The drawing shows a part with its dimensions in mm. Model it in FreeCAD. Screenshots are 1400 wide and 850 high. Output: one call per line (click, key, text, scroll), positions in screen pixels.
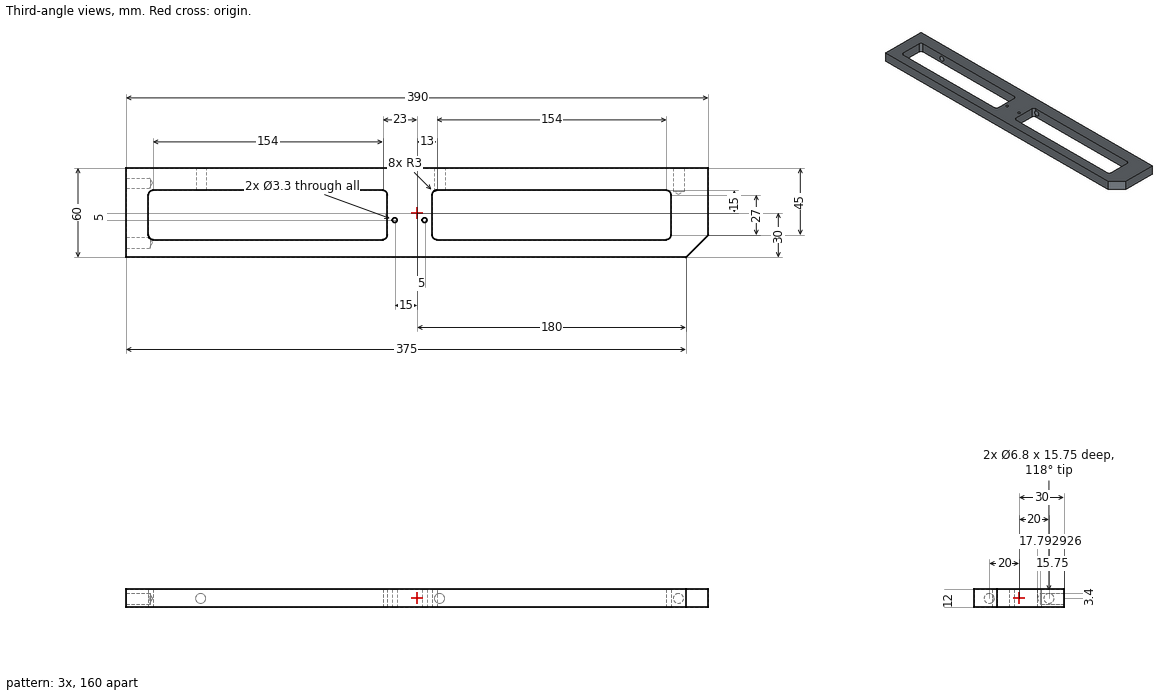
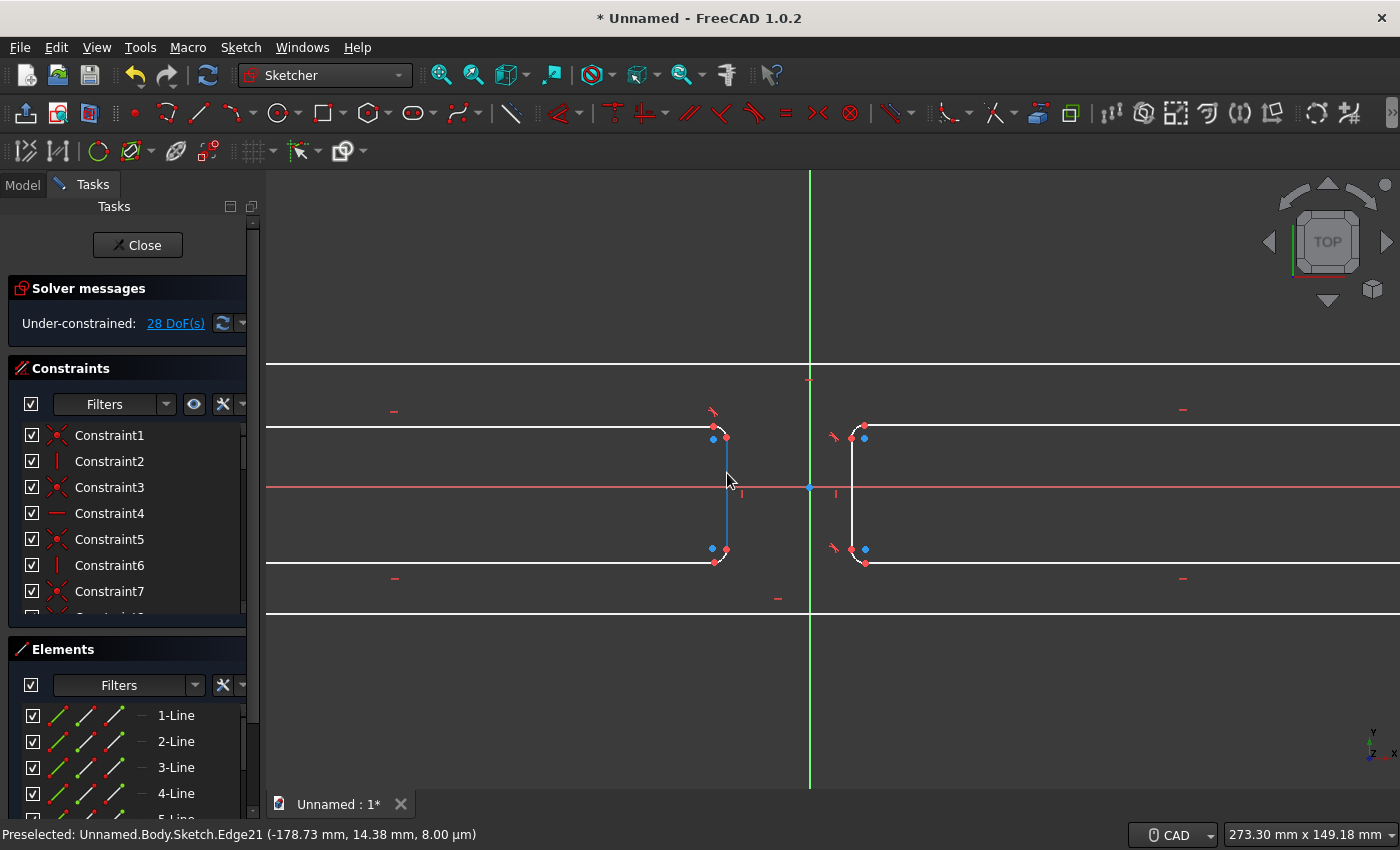
click(727, 471)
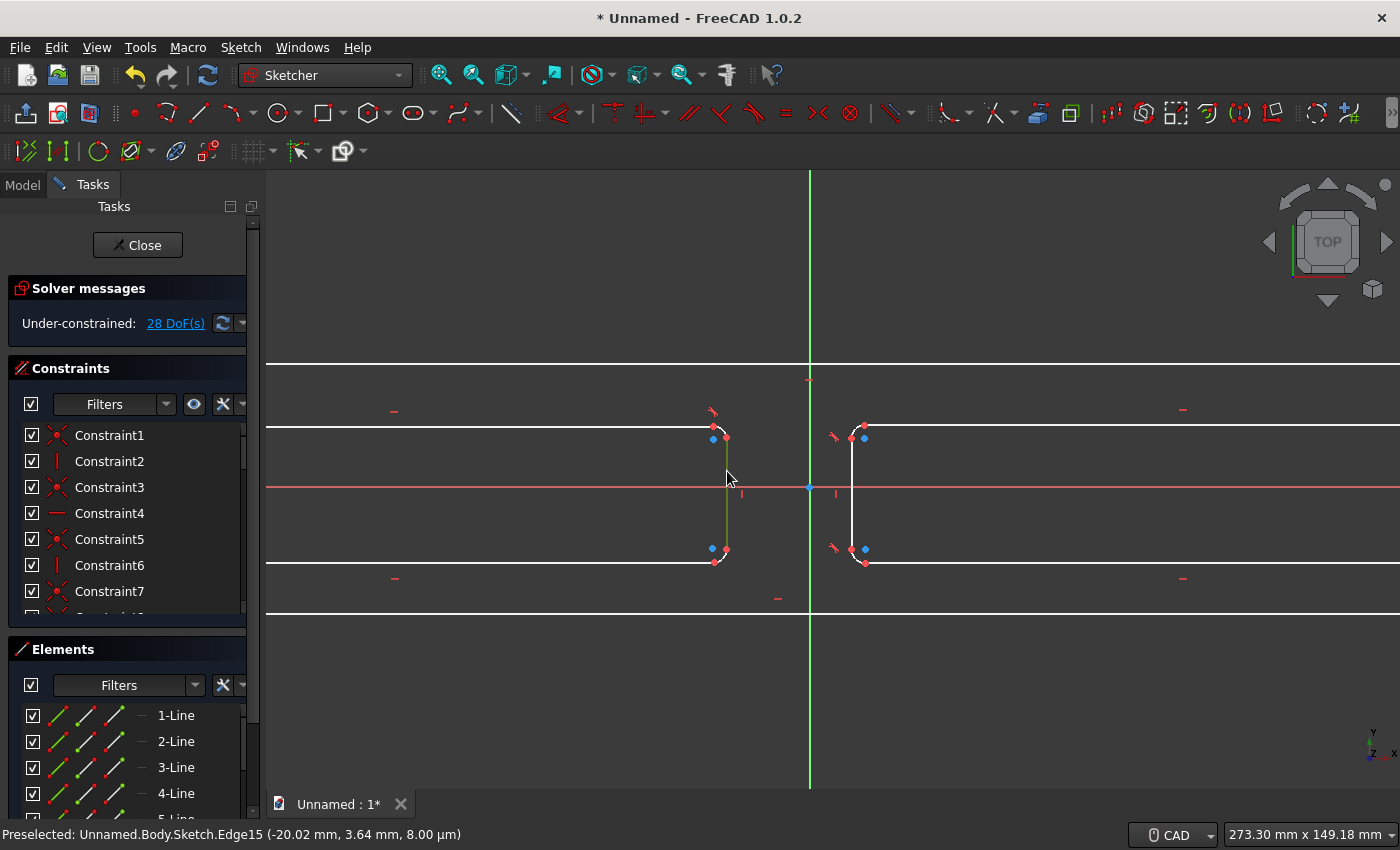
scroll(723, 430, up, 3)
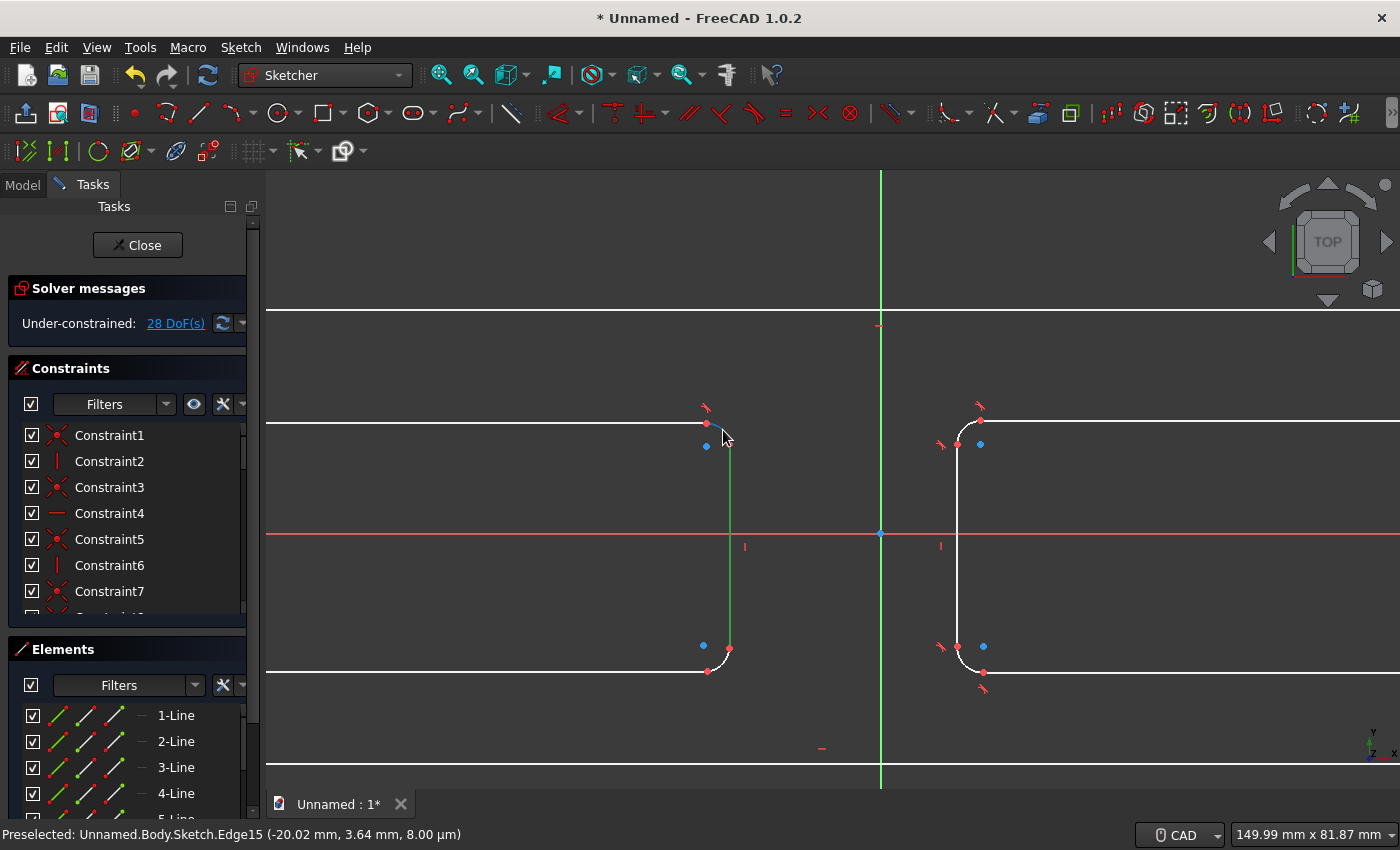
click(722, 429)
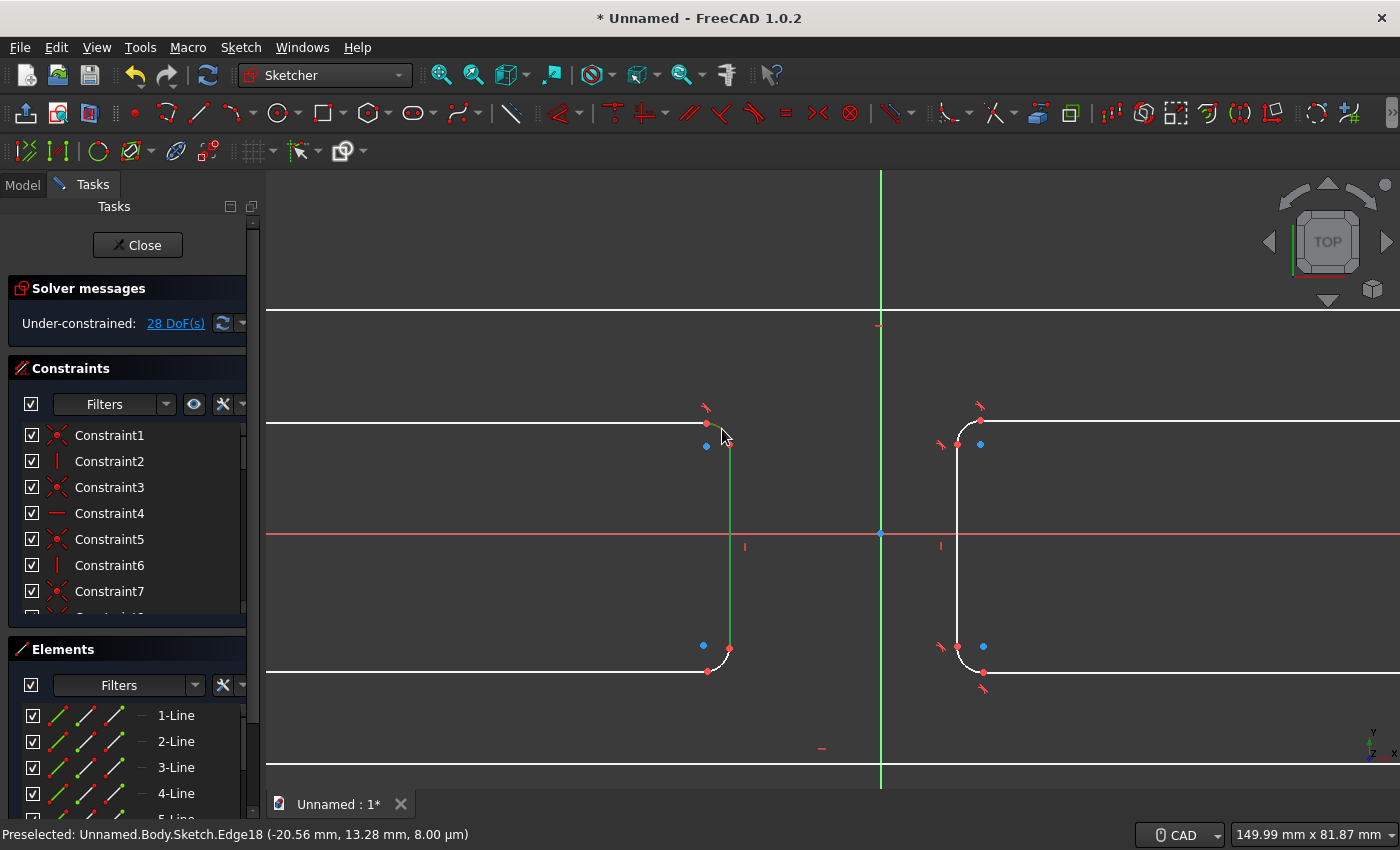
key(t)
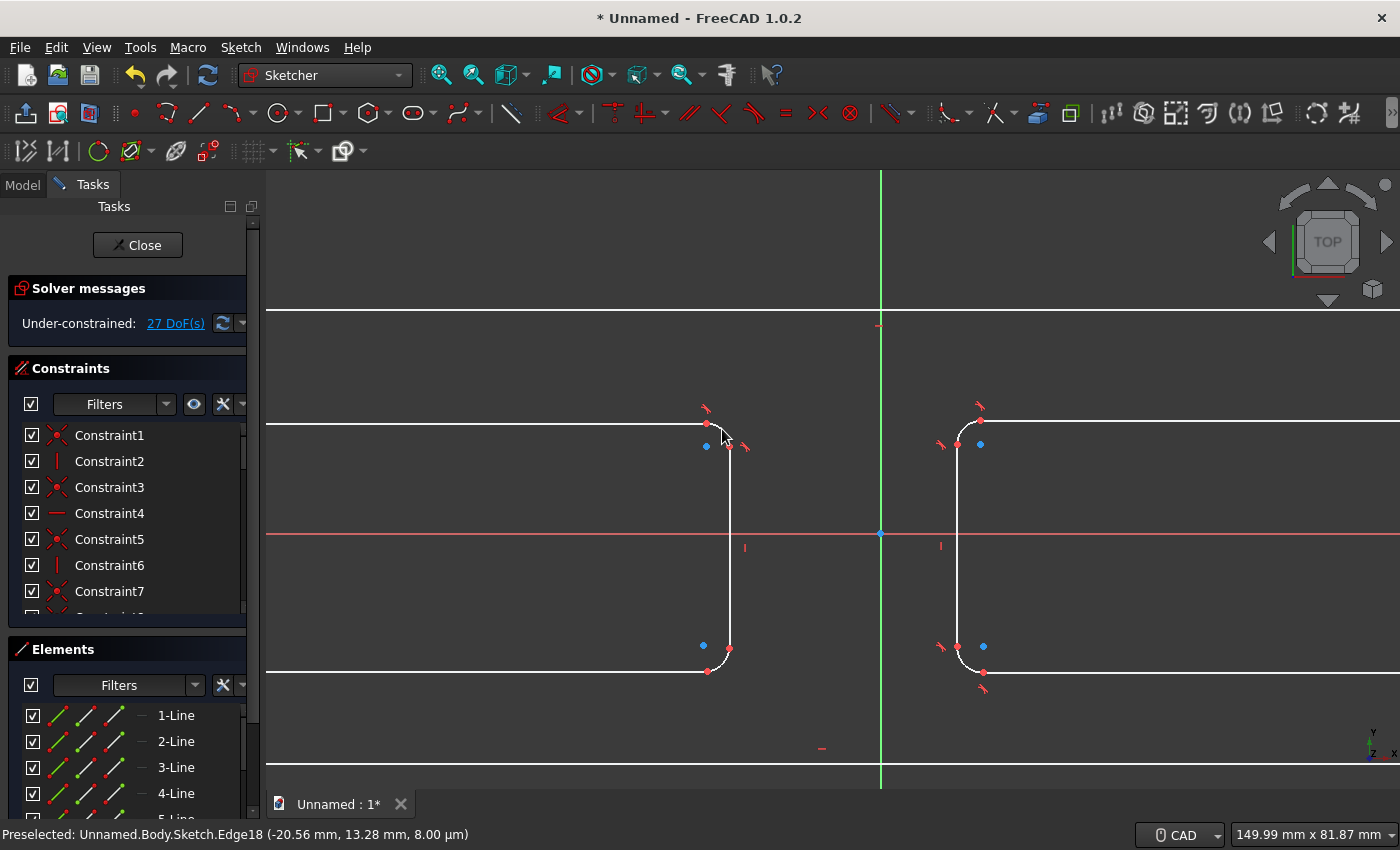
click(730, 507)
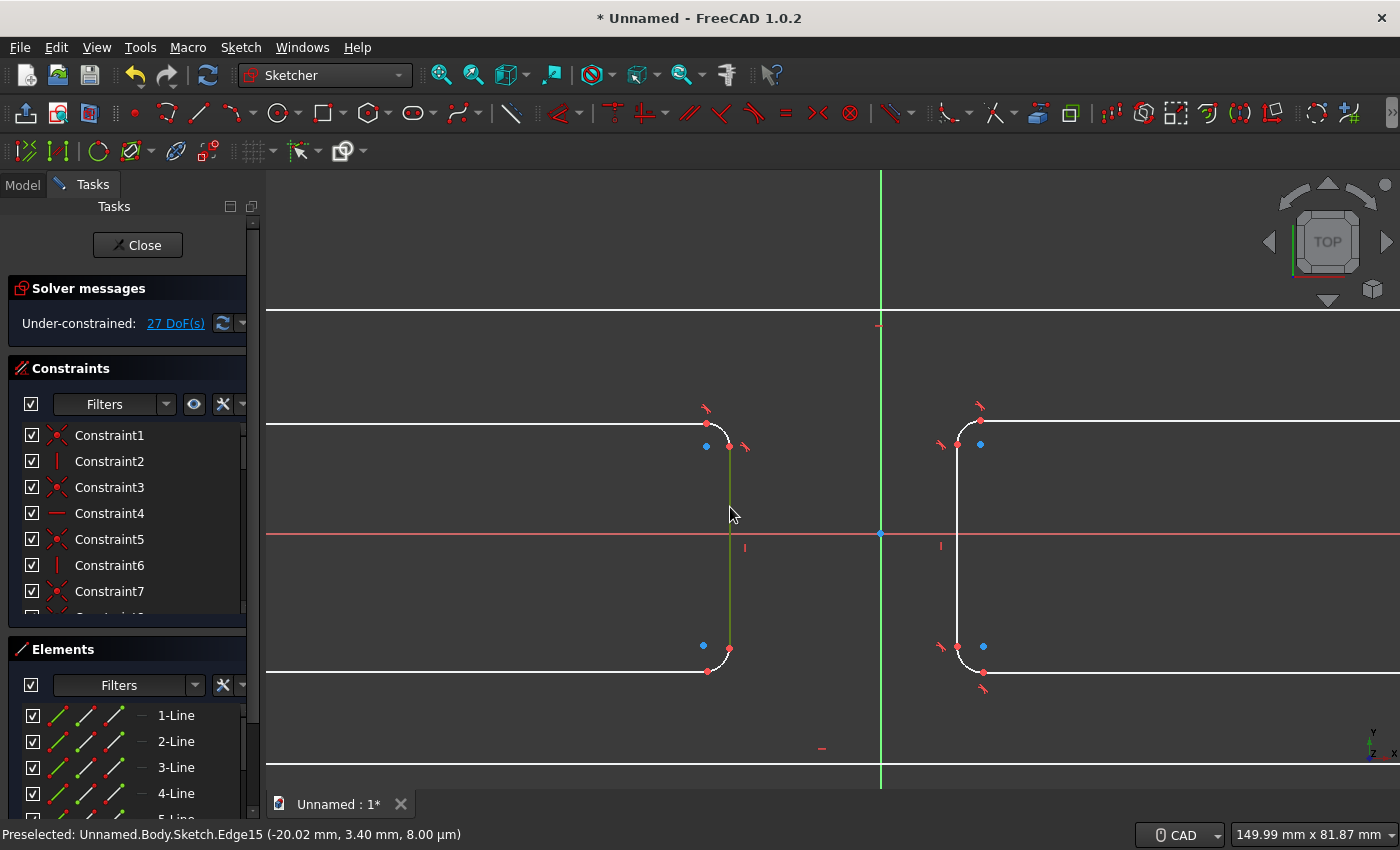
scroll(717, 668, up, 2)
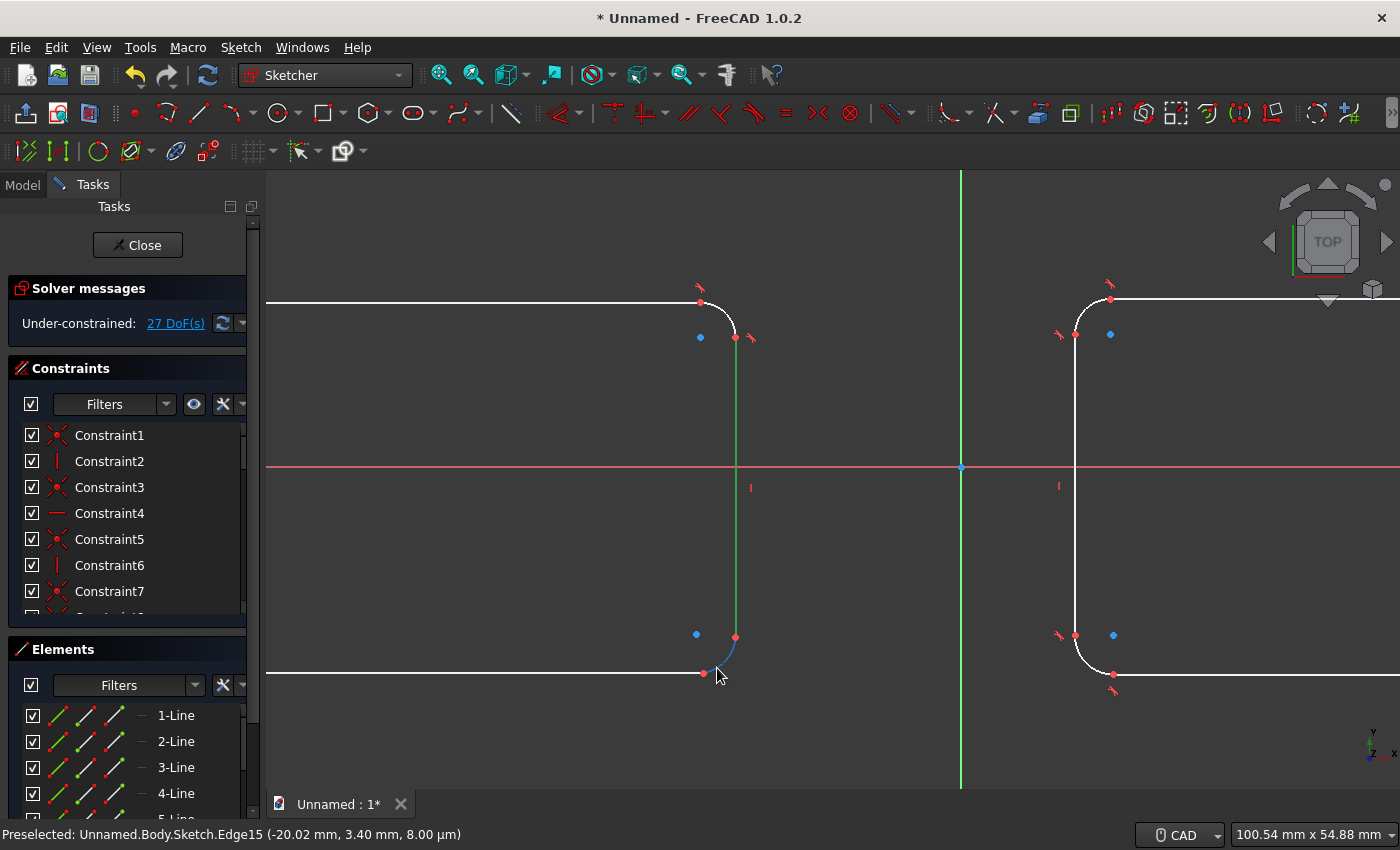
click(717, 668)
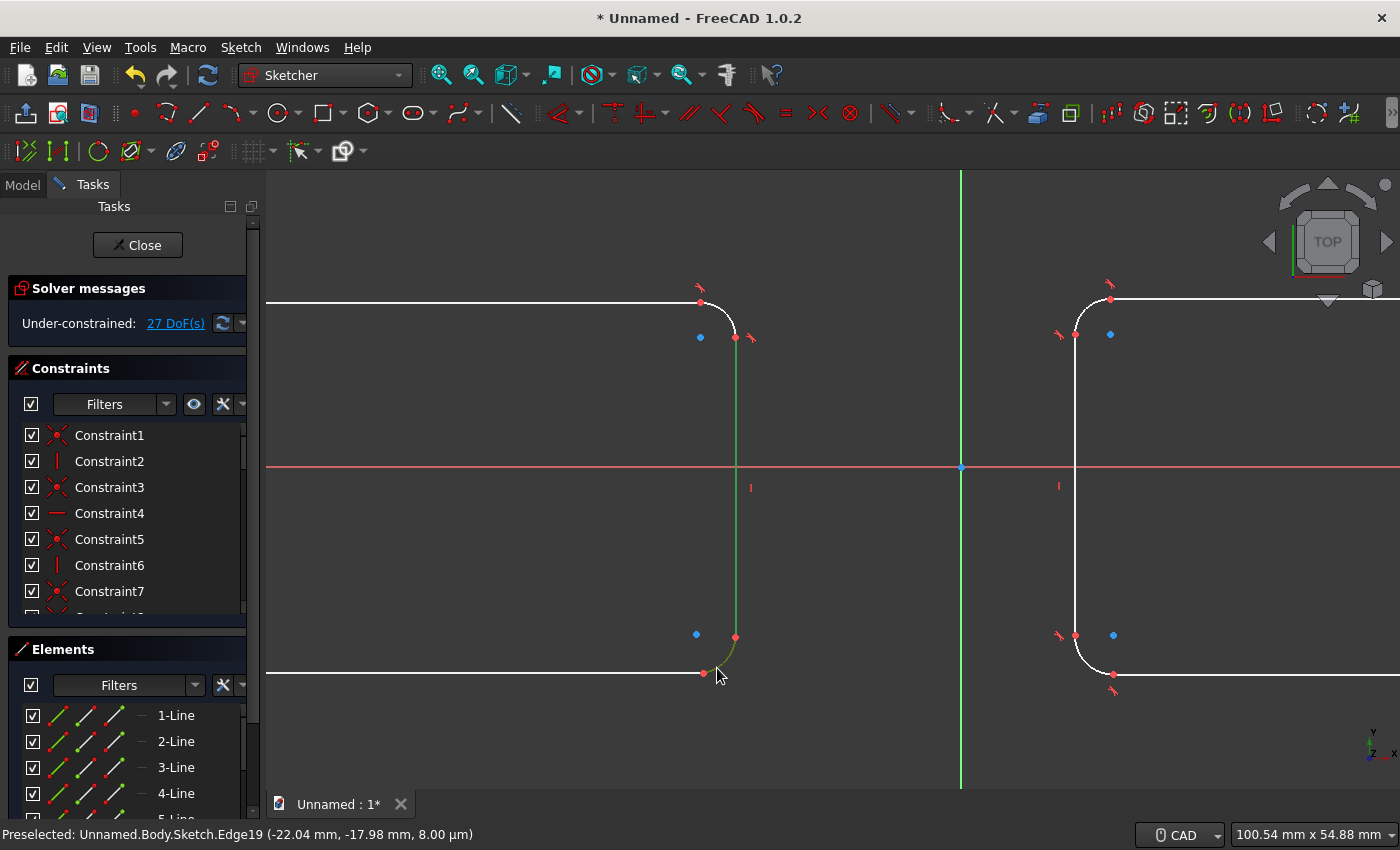
click(754, 114)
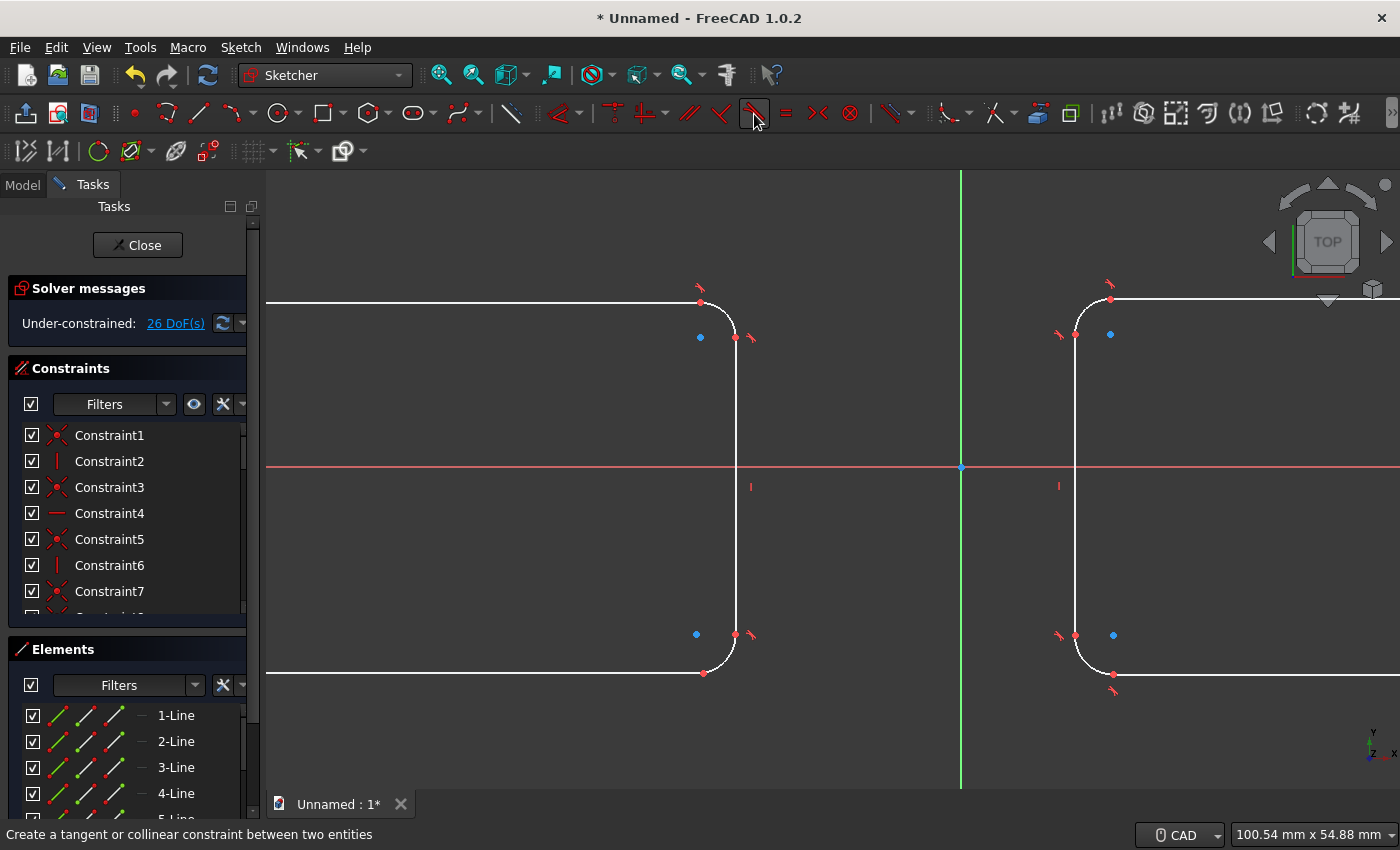
scroll(726, 482, down, 9)